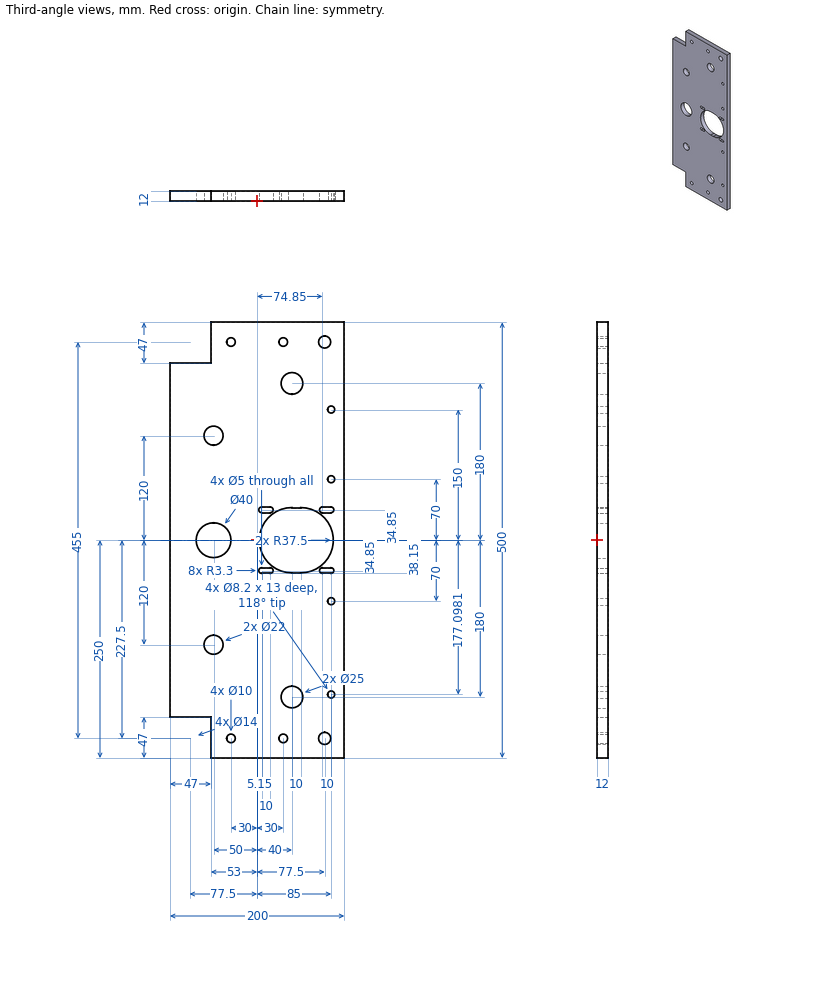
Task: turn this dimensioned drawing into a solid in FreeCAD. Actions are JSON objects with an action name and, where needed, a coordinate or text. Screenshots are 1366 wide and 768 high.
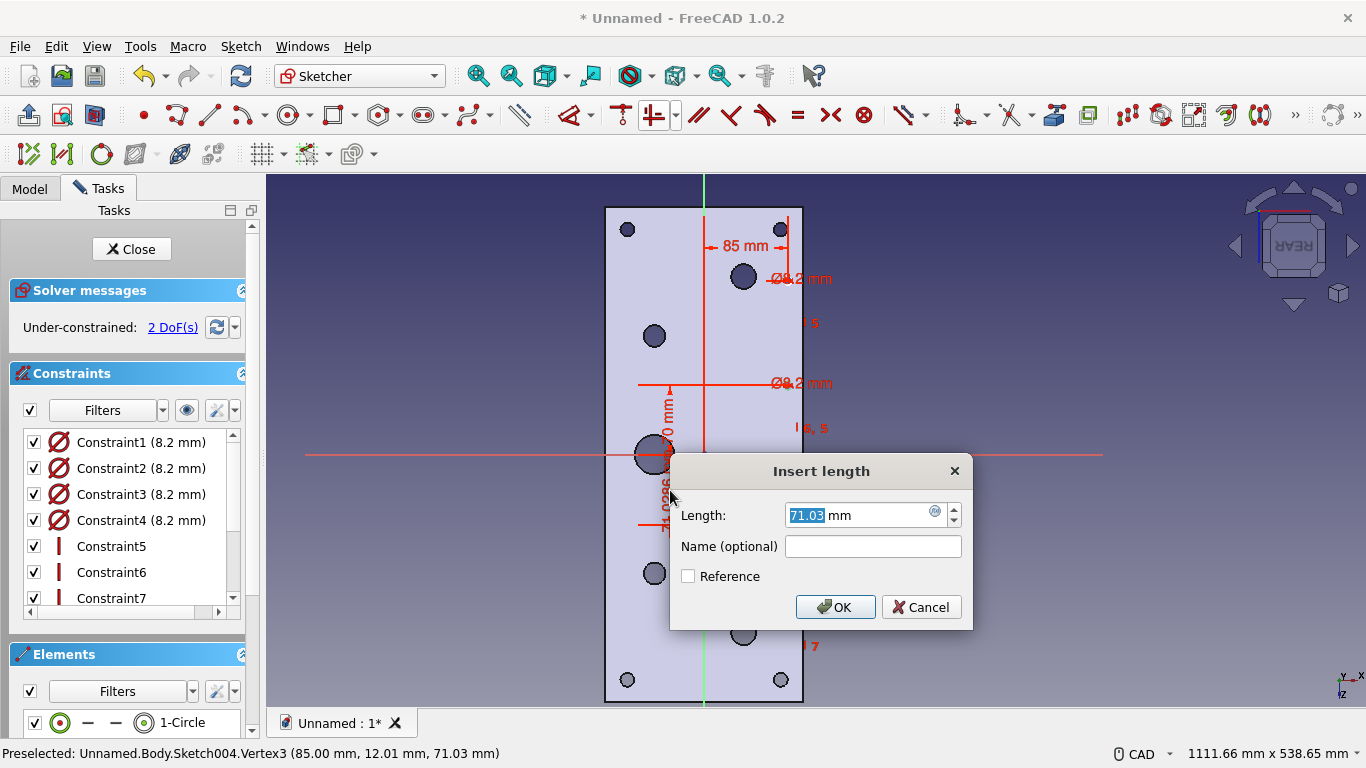
{"action": "type", "text": "70"}
{"action": "key", "text": "Return"}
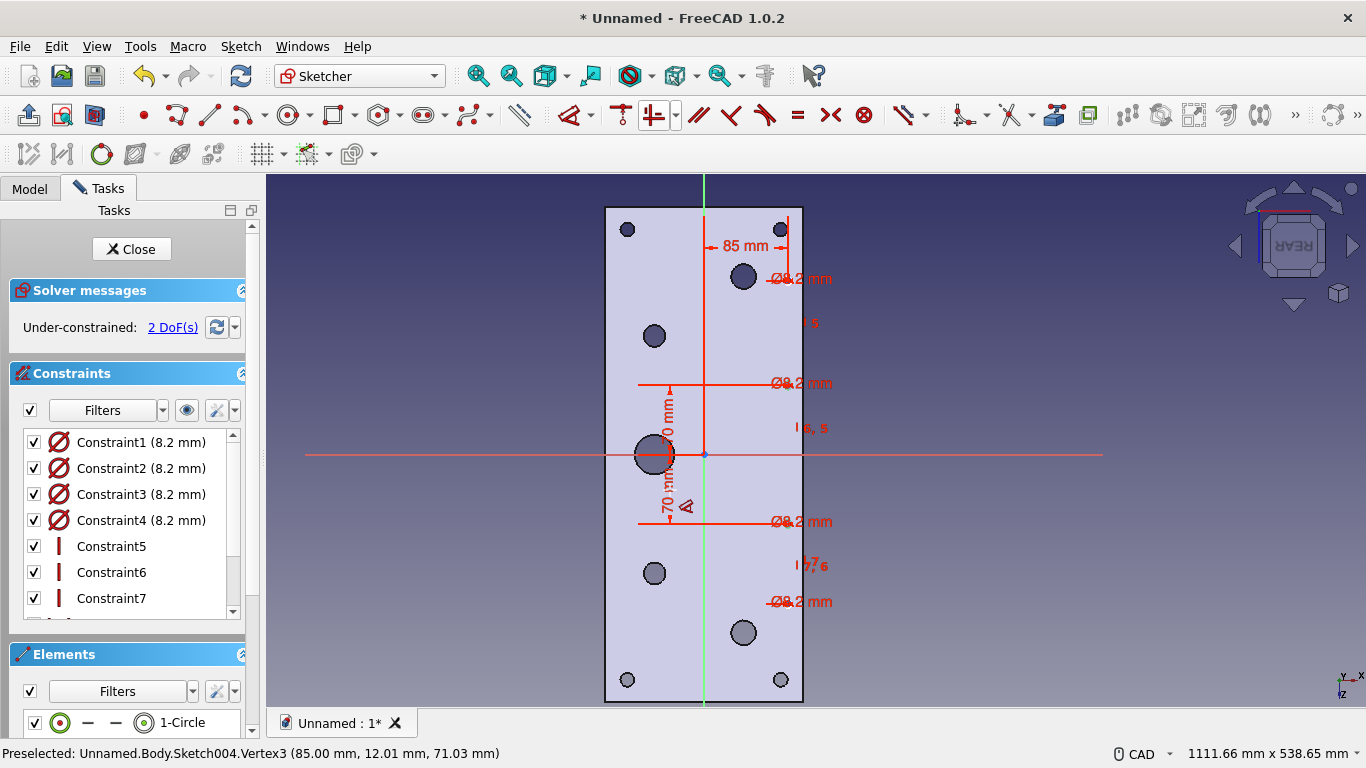
{"action": "left_click", "coordinate": [788, 604]}
{"action": "left_click", "coordinate": [670, 529]}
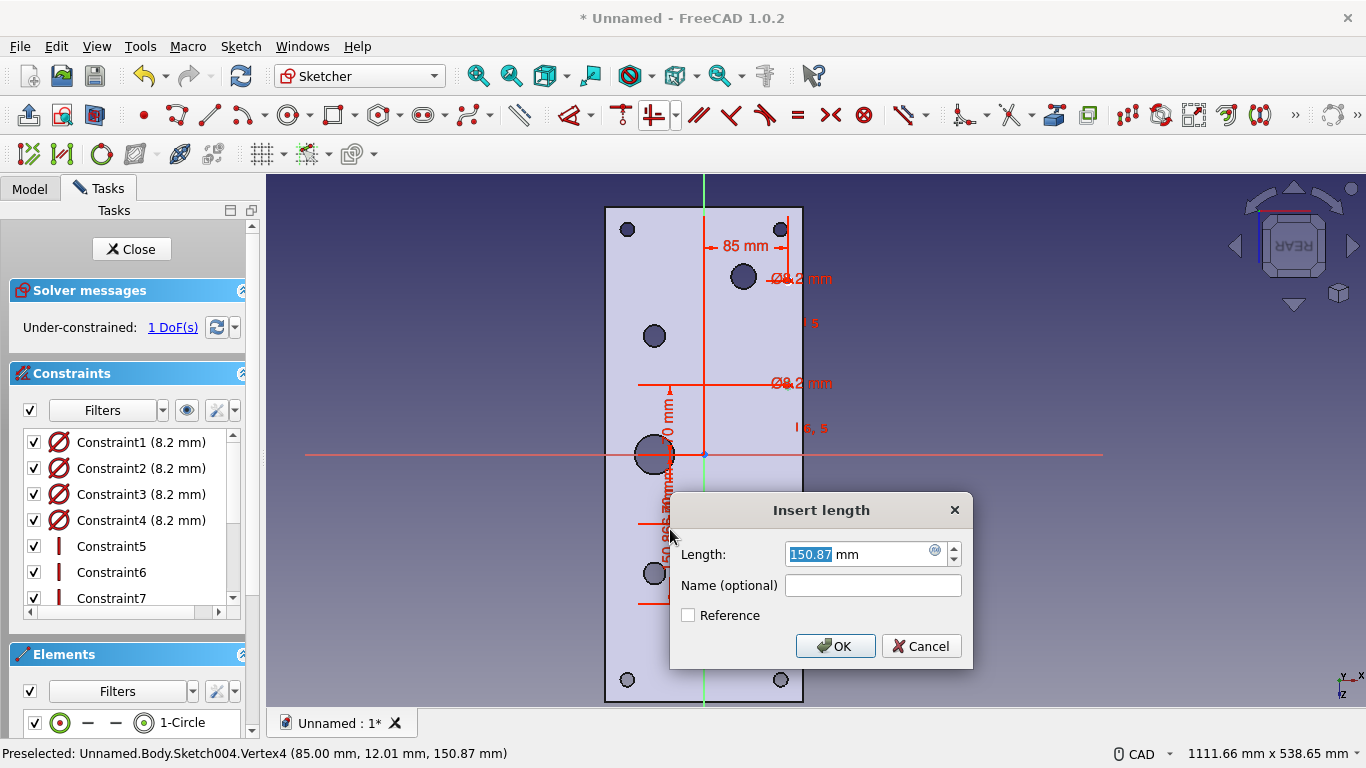
{"action": "type", "text": "150"}
{"action": "key", "text": "Return"}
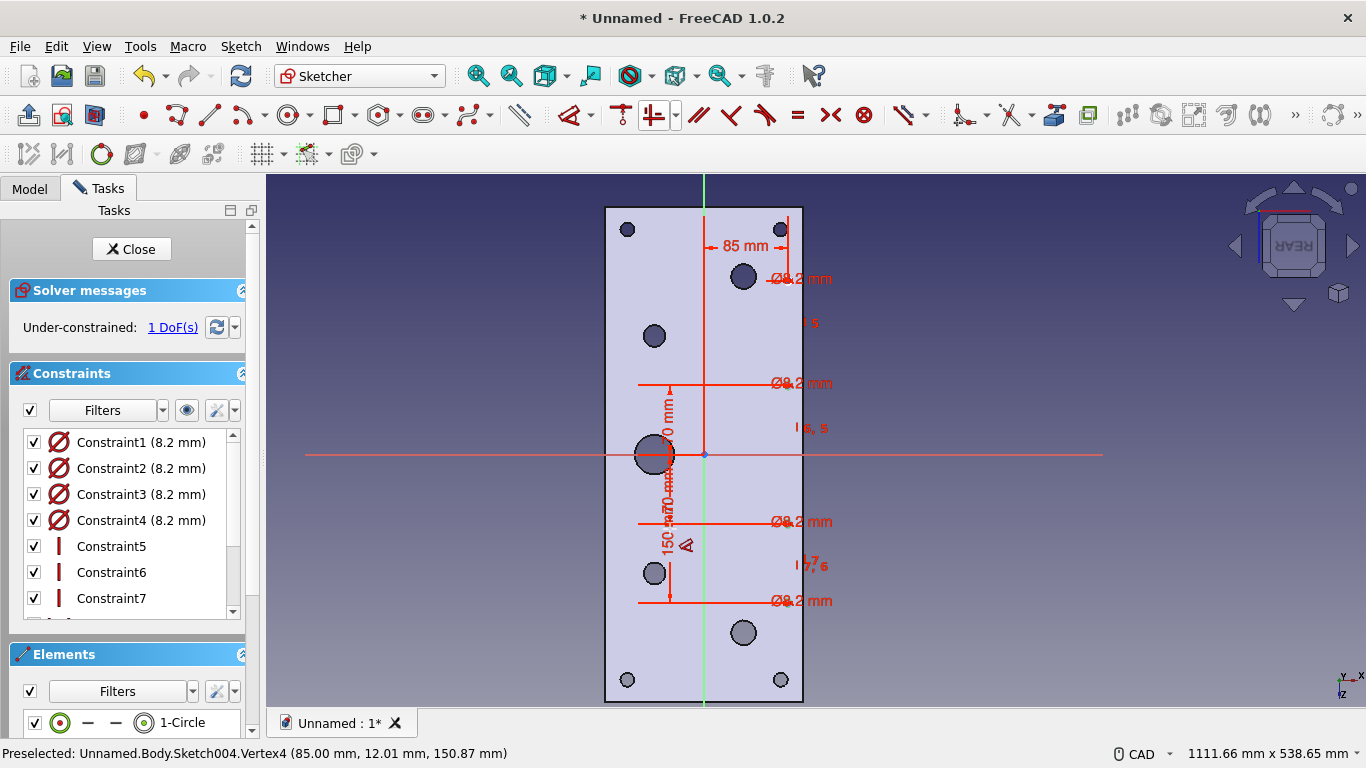
{"action": "left_click", "coordinate": [788, 281]}
{"action": "left_click", "coordinate": [670, 368]}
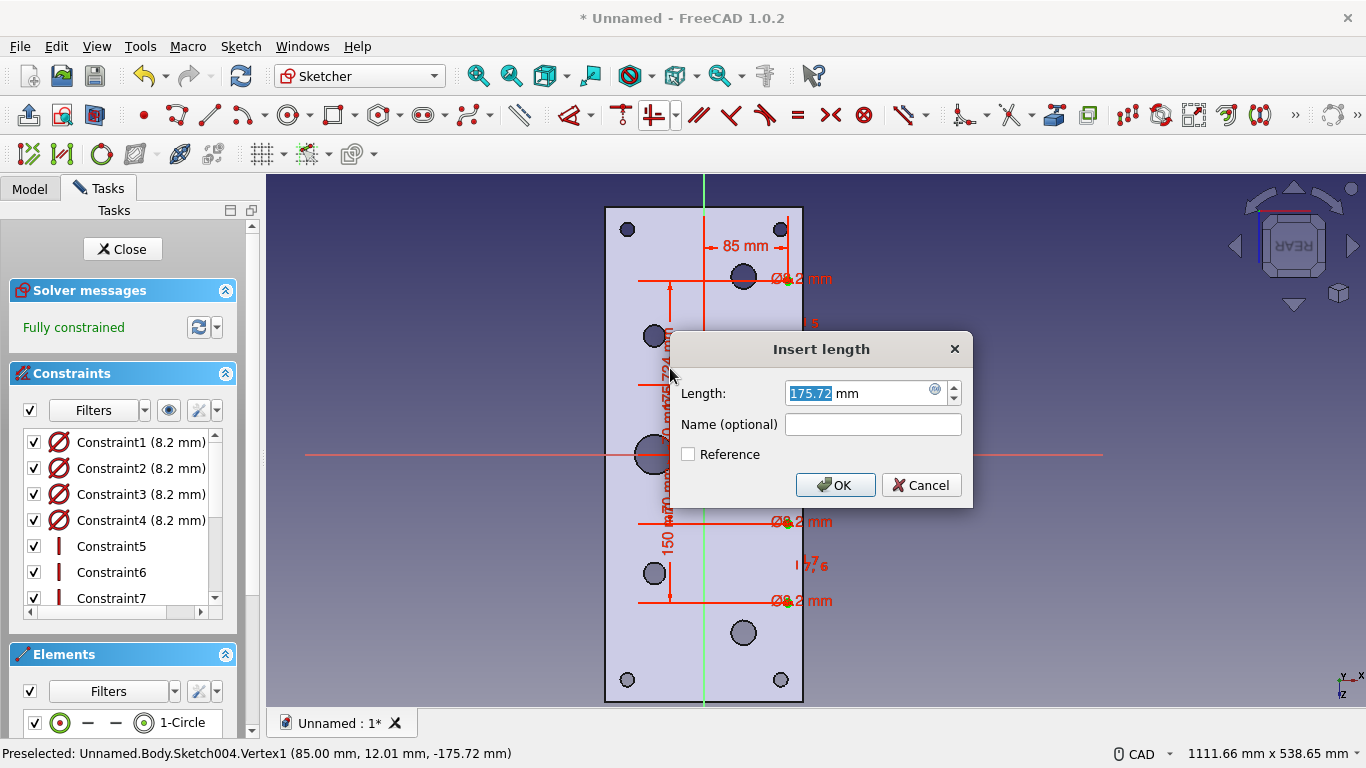
{"action": "type", "text": "177.0981"}
{"action": "key", "text": "Return"}
{"action": "key", "text": "Escape"}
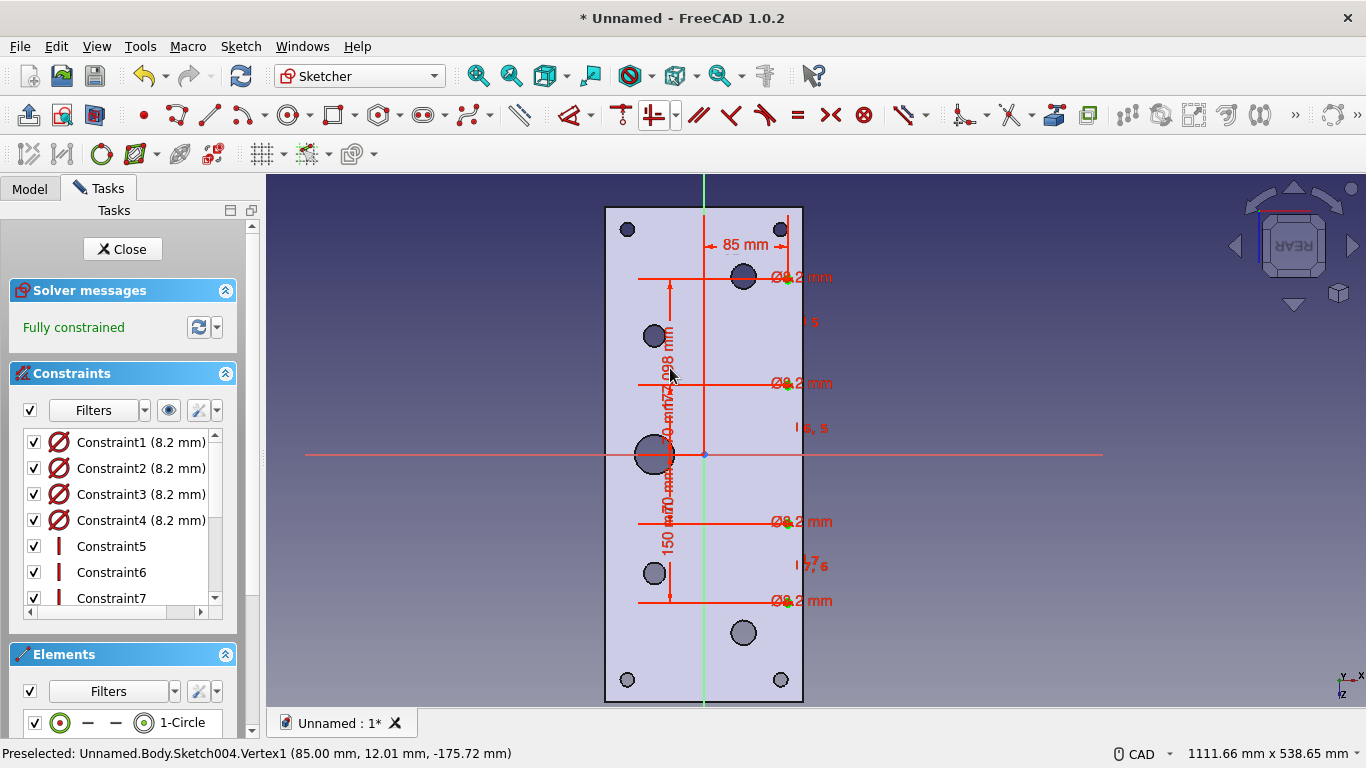
{"action": "left_click", "coordinate": [123, 249]}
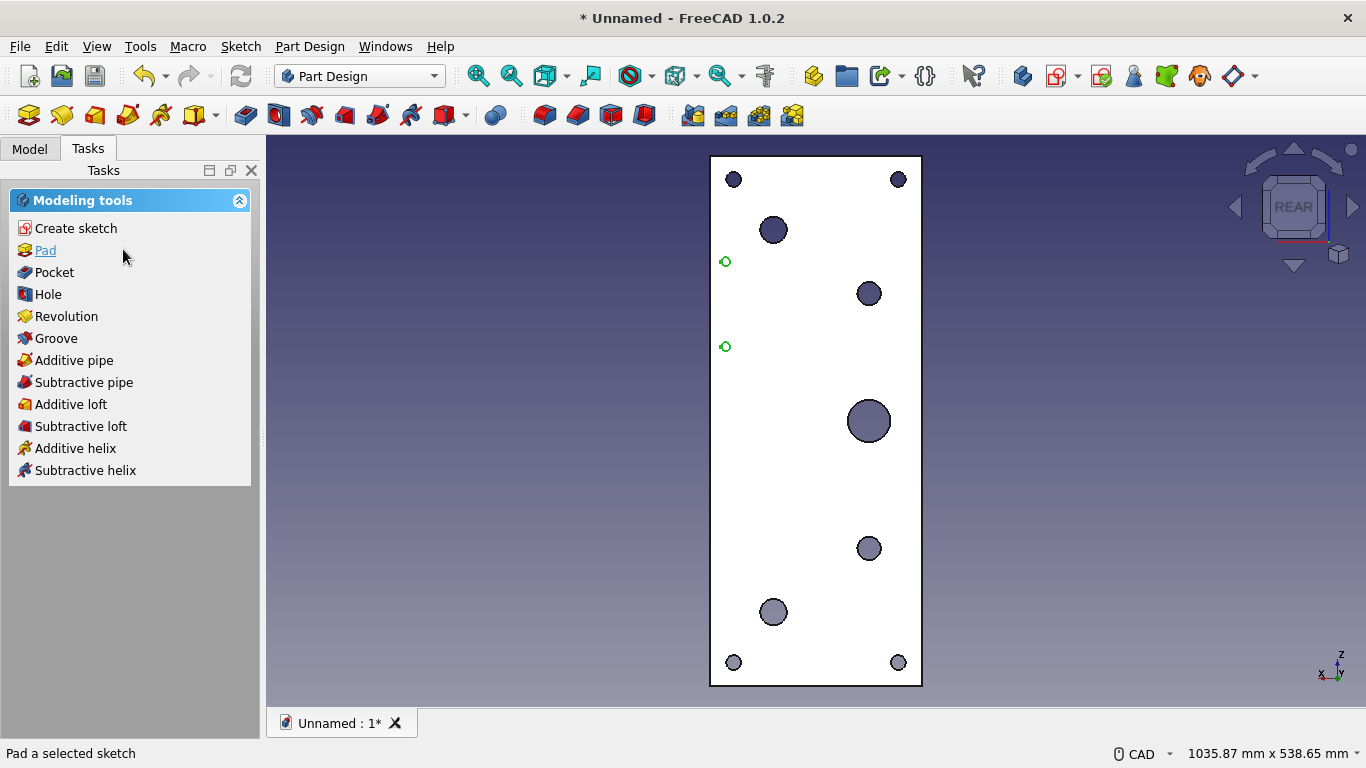
{"action": "left_click", "coordinate": [279, 116]}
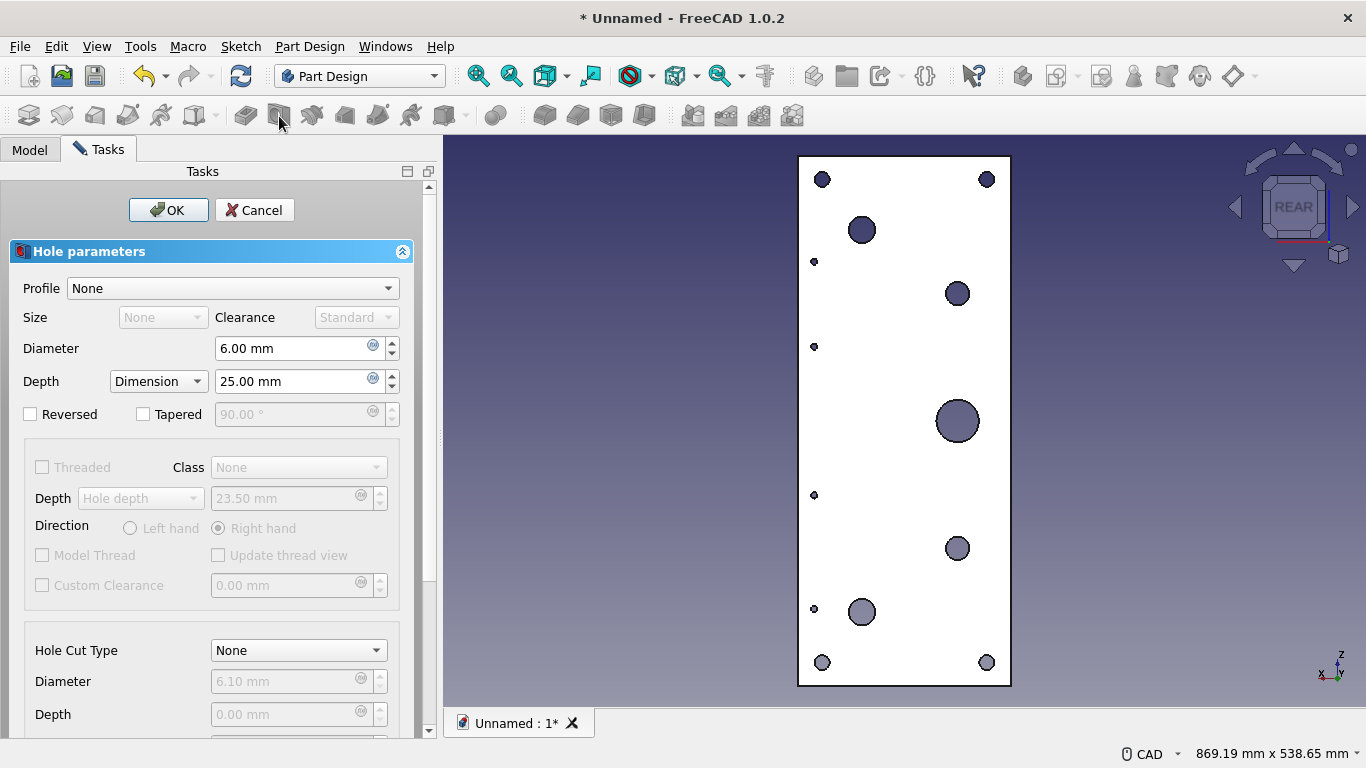
{"action": "triple_click", "coordinate": [300, 348]}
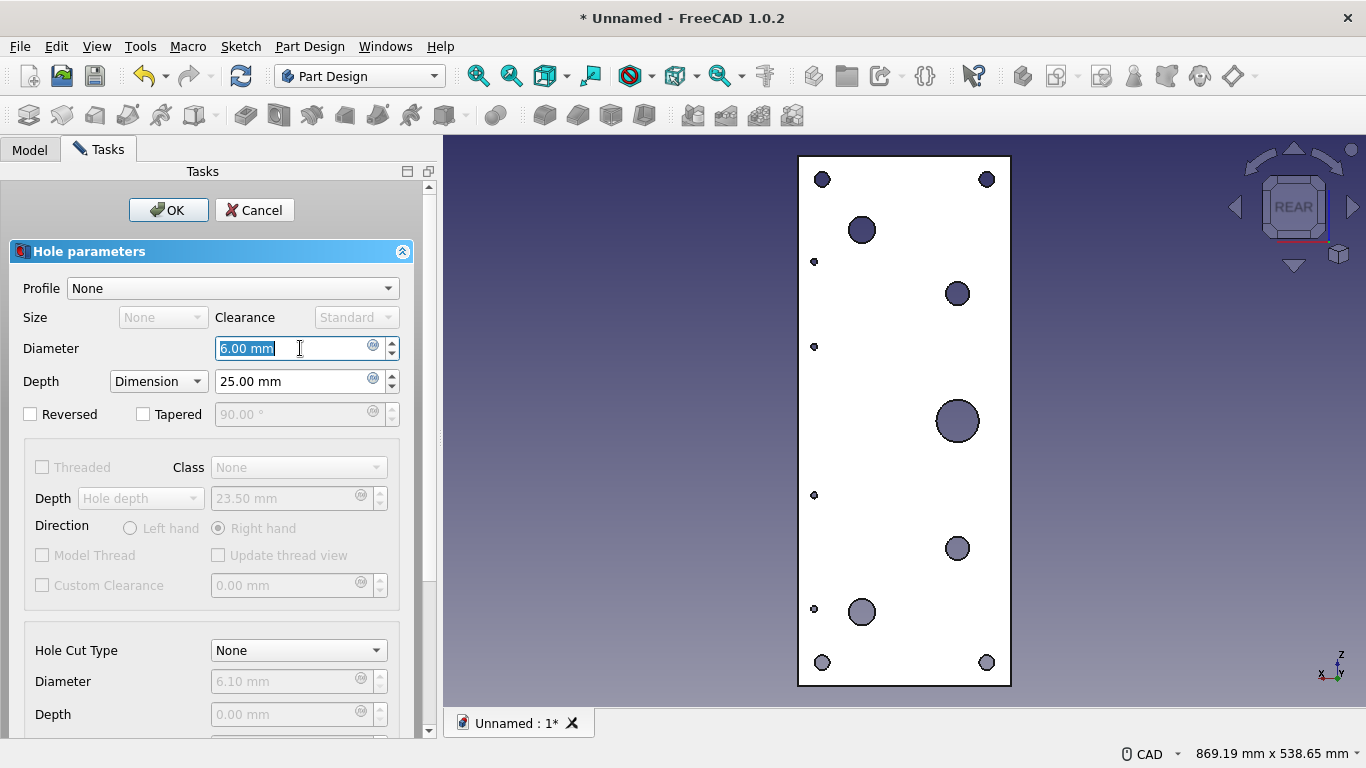
{"action": "type", "text": "8.2"}
{"action": "key", "text": "Tab"}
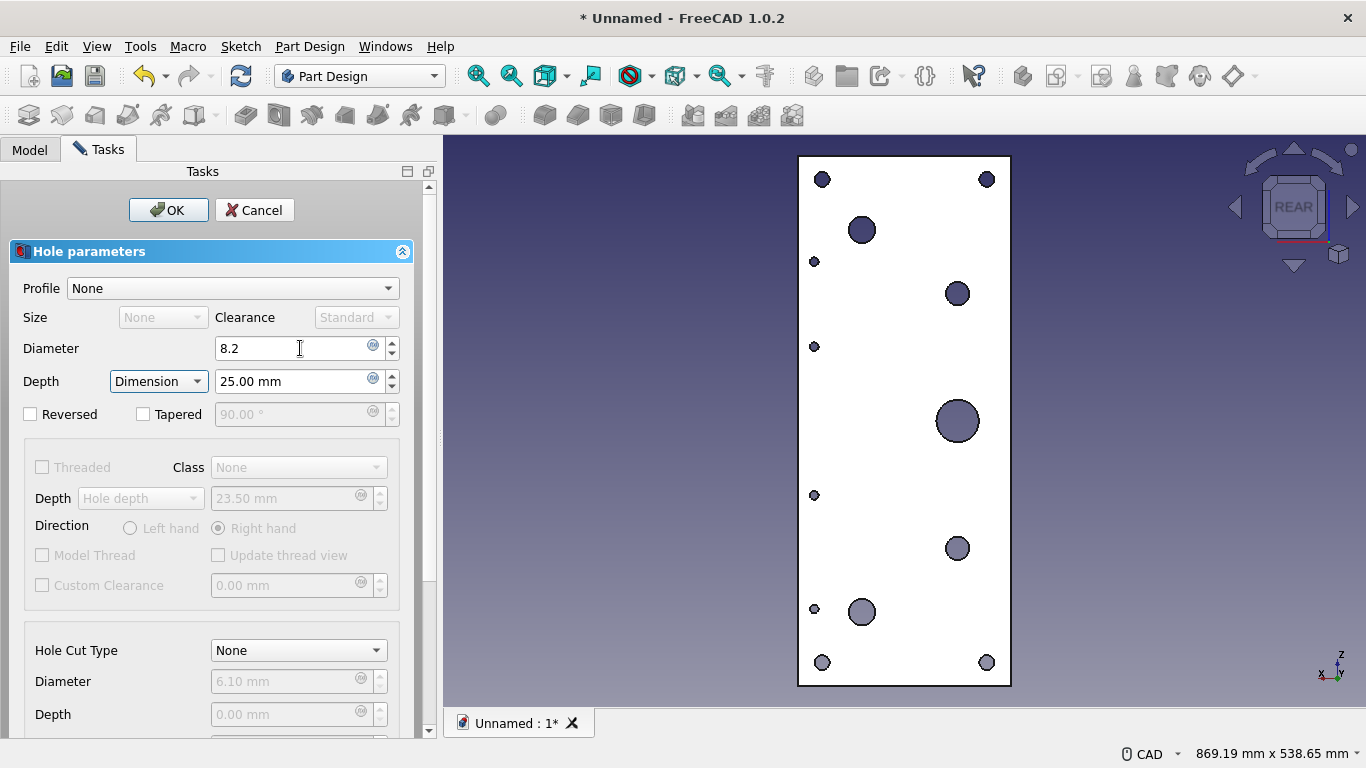
{"action": "triple_click", "coordinate": [300, 382]}